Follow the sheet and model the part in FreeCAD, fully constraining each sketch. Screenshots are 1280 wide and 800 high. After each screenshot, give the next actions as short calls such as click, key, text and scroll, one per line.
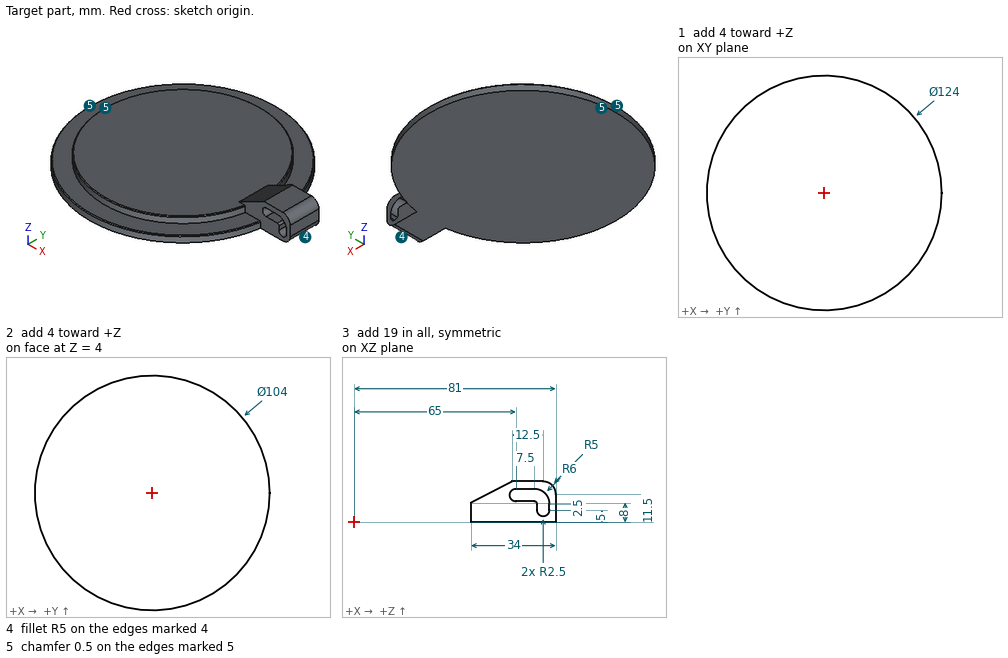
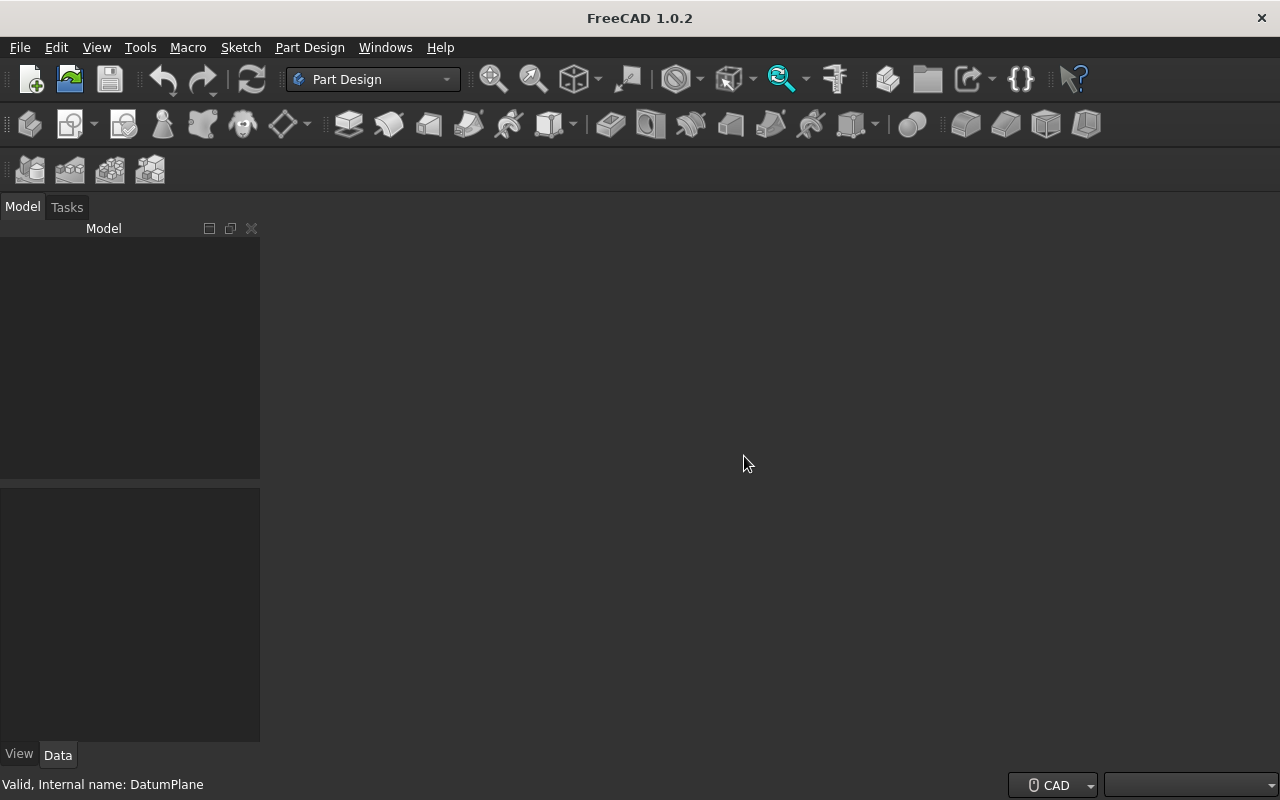
click(30, 80)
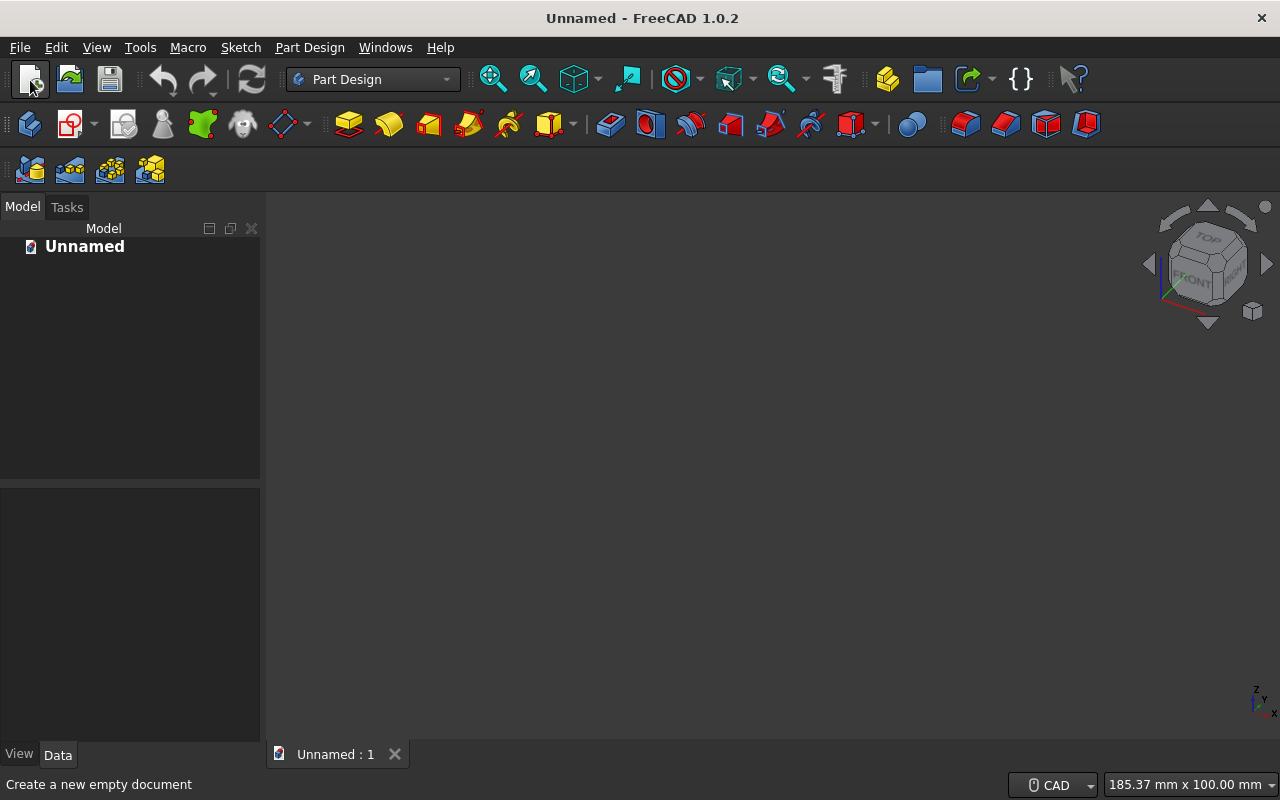
click(70, 124)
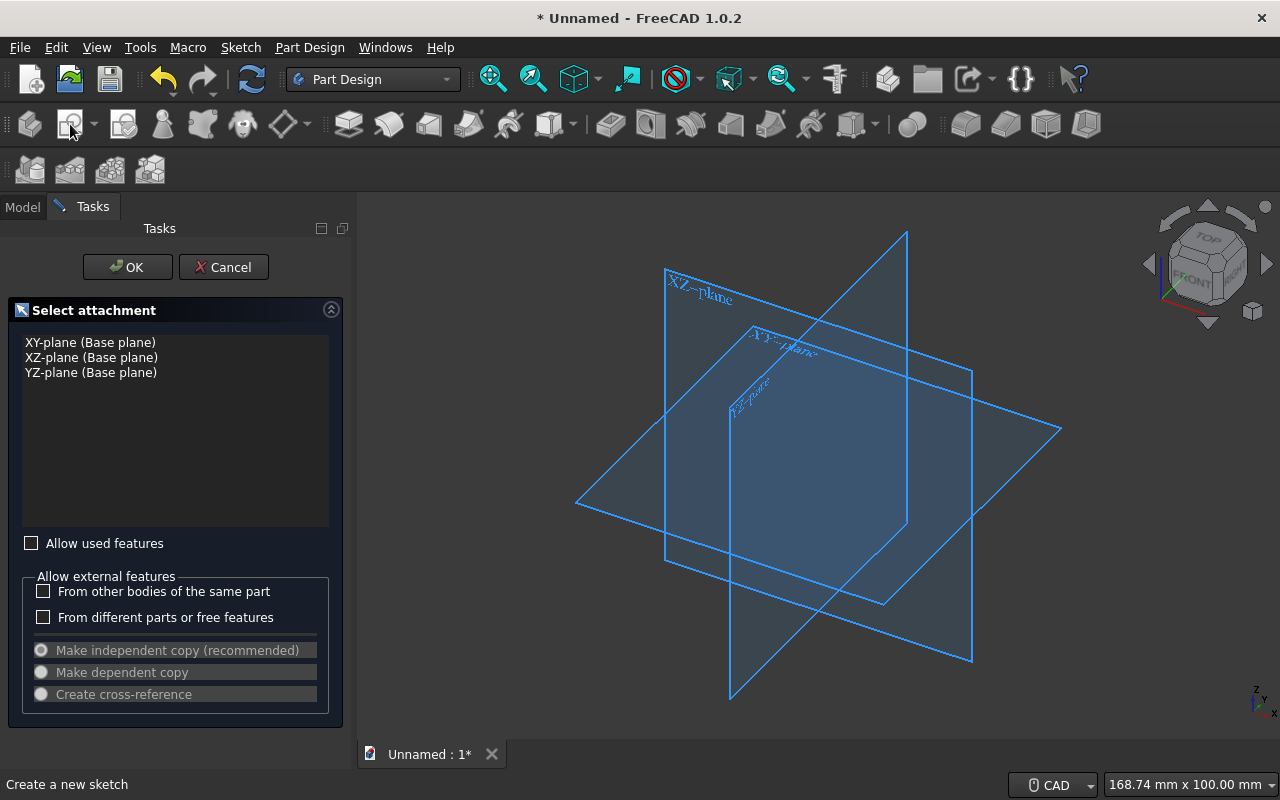
click(82, 342)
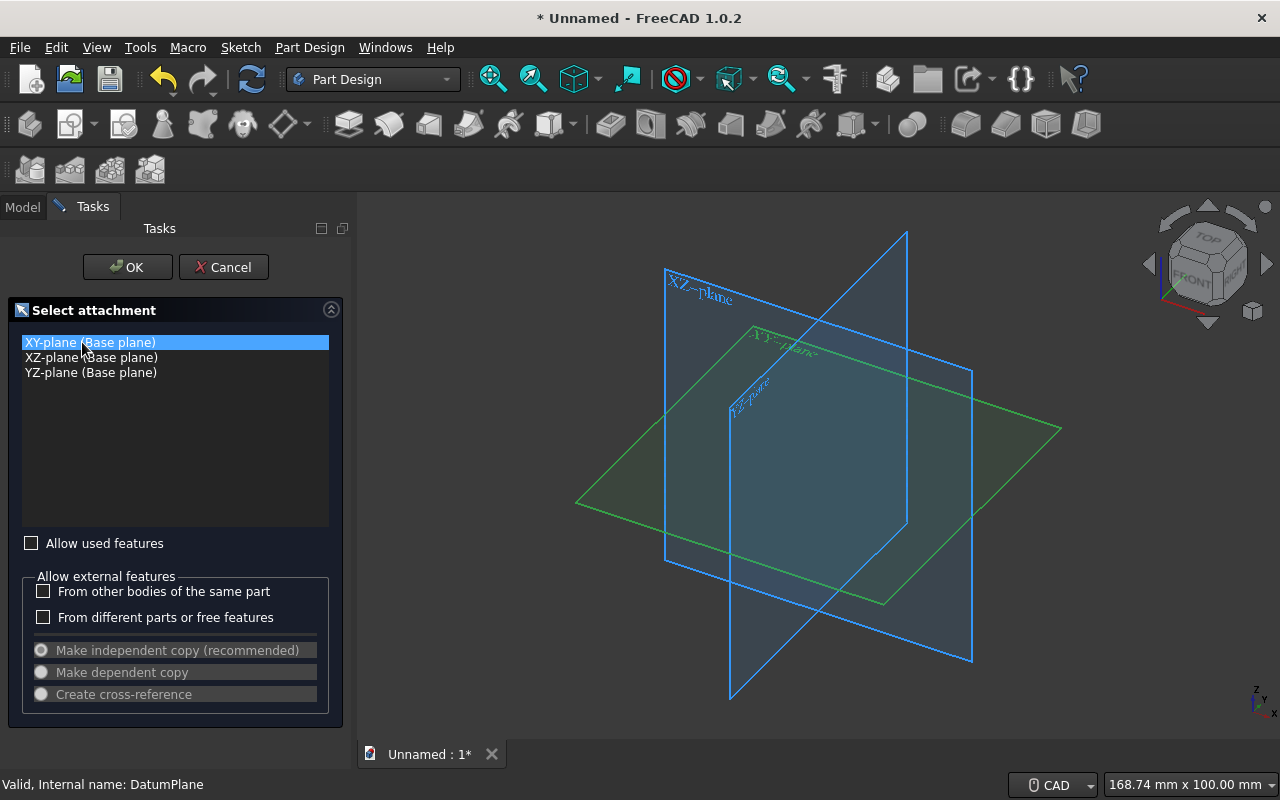
click(128, 267)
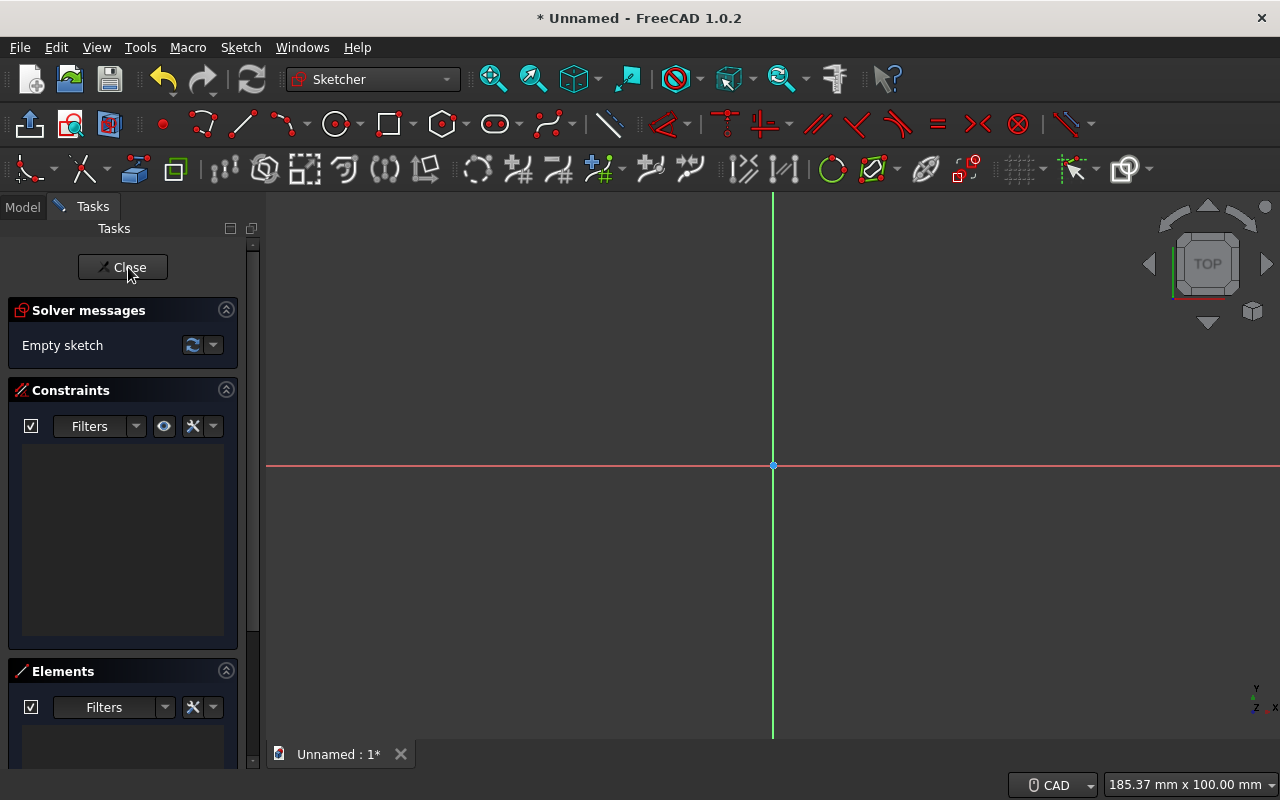
scroll(621, 466, down, 3)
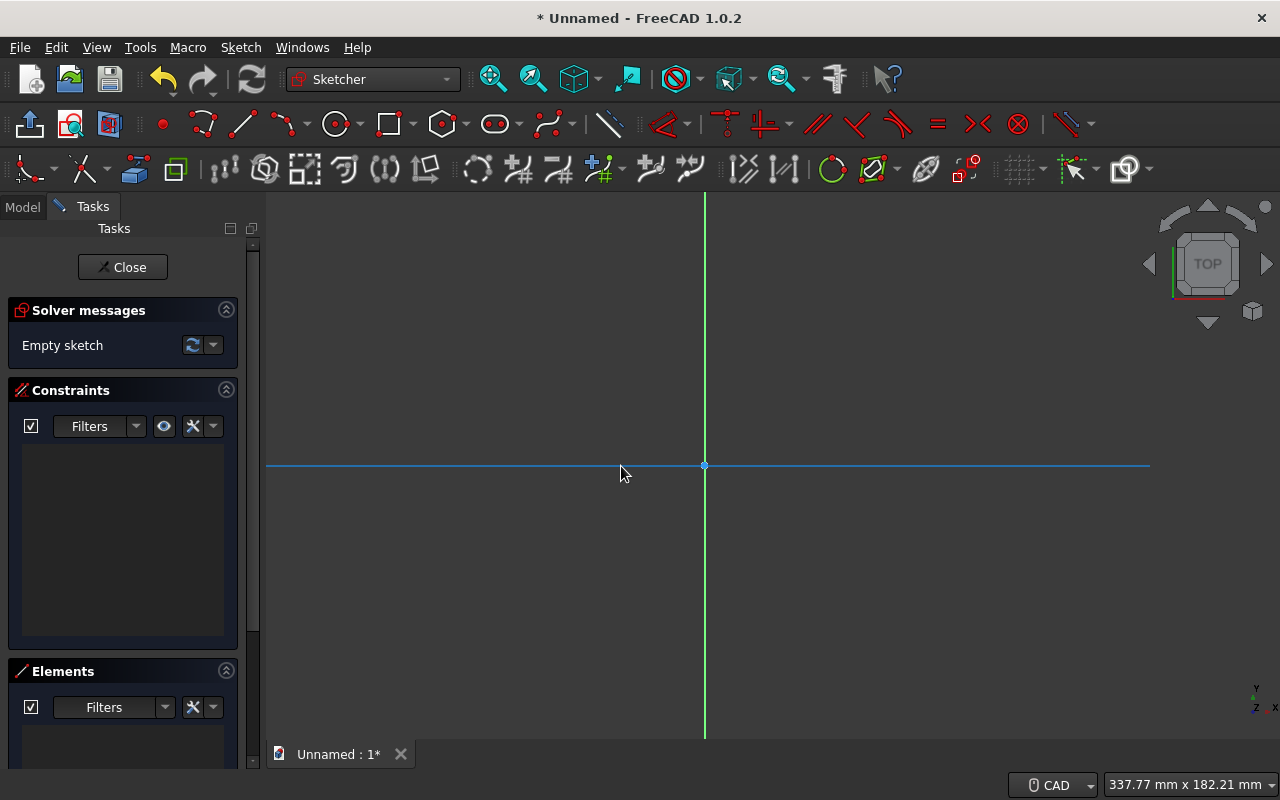
click(336, 124)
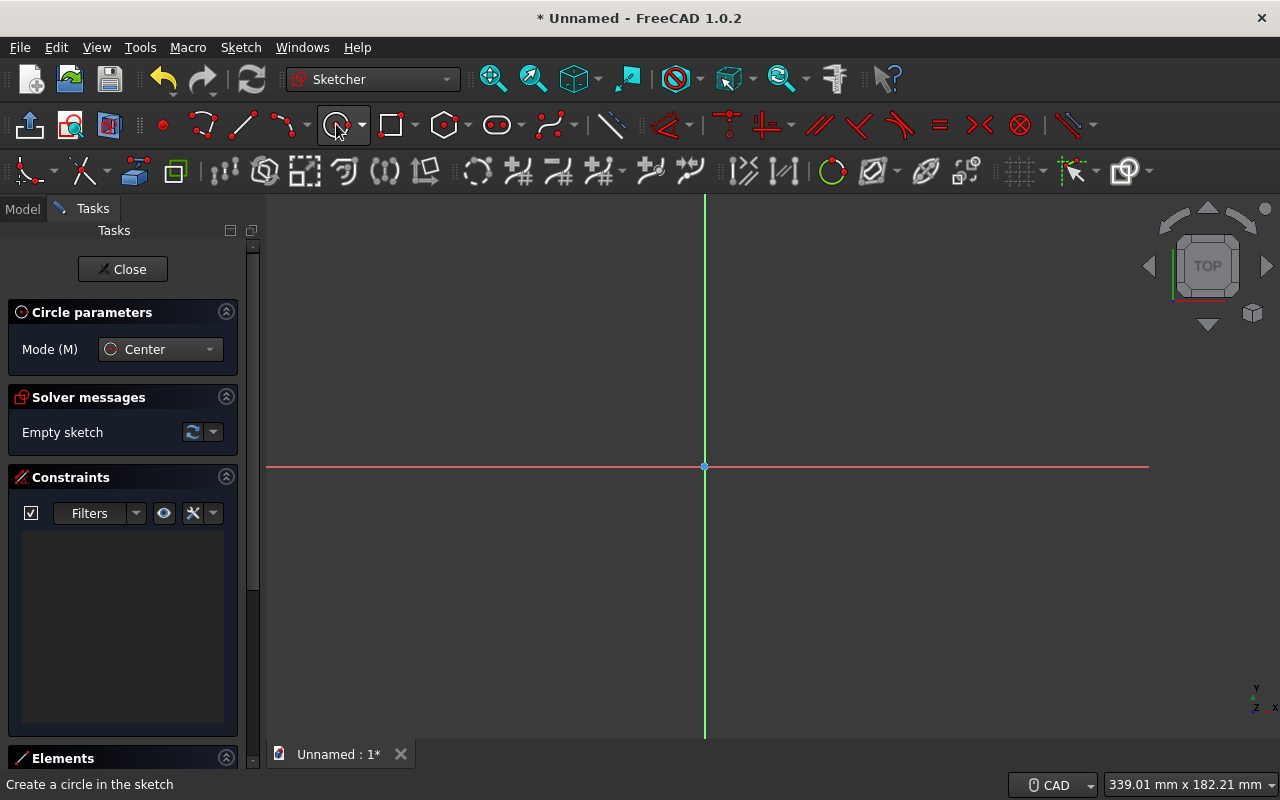
click(705, 467)
click(836, 336)
key(Escape)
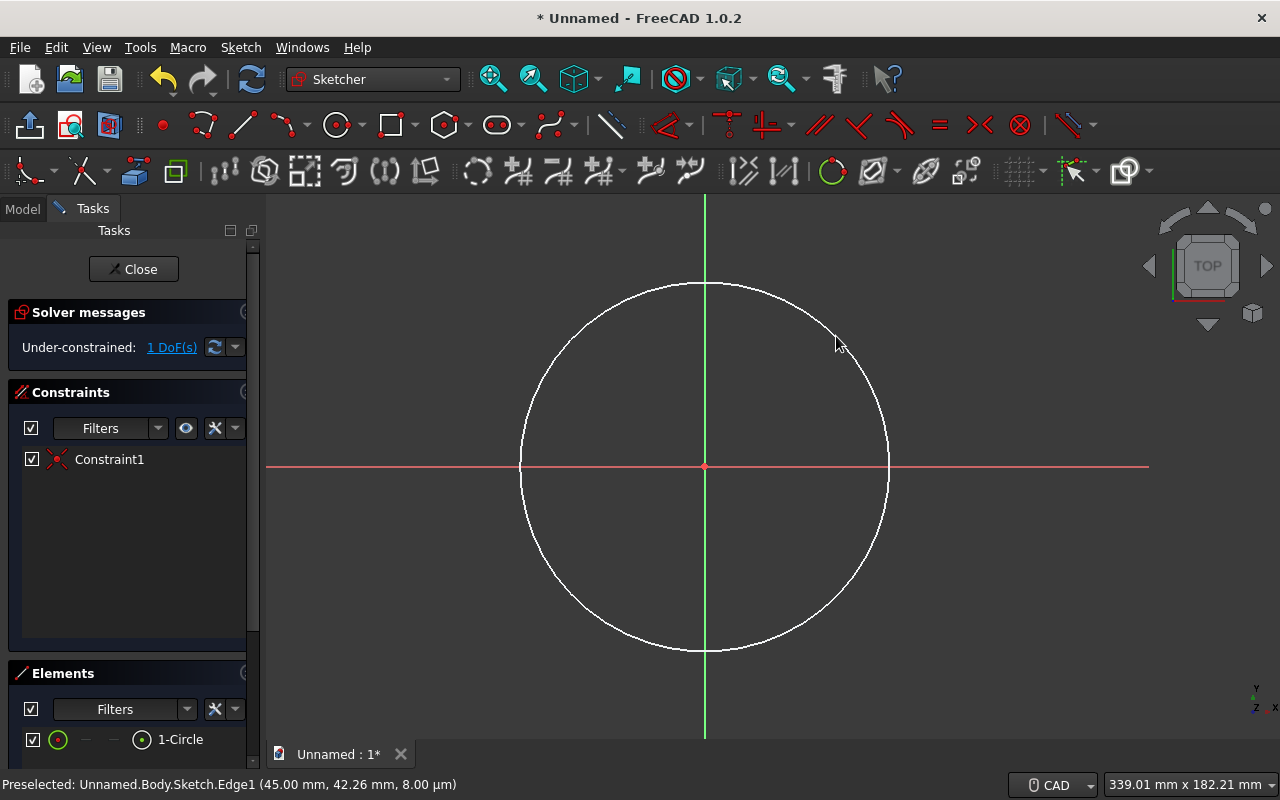
click(835, 336)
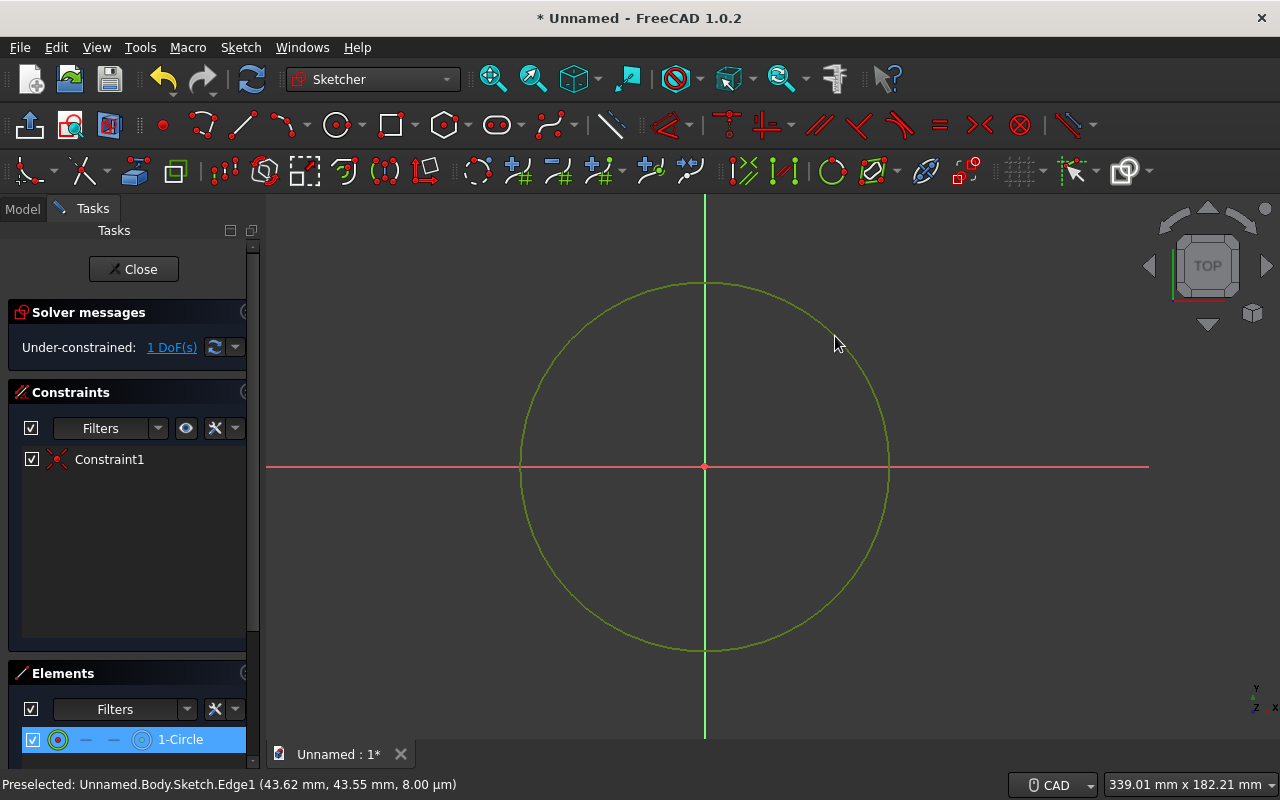
key(k)
key(o)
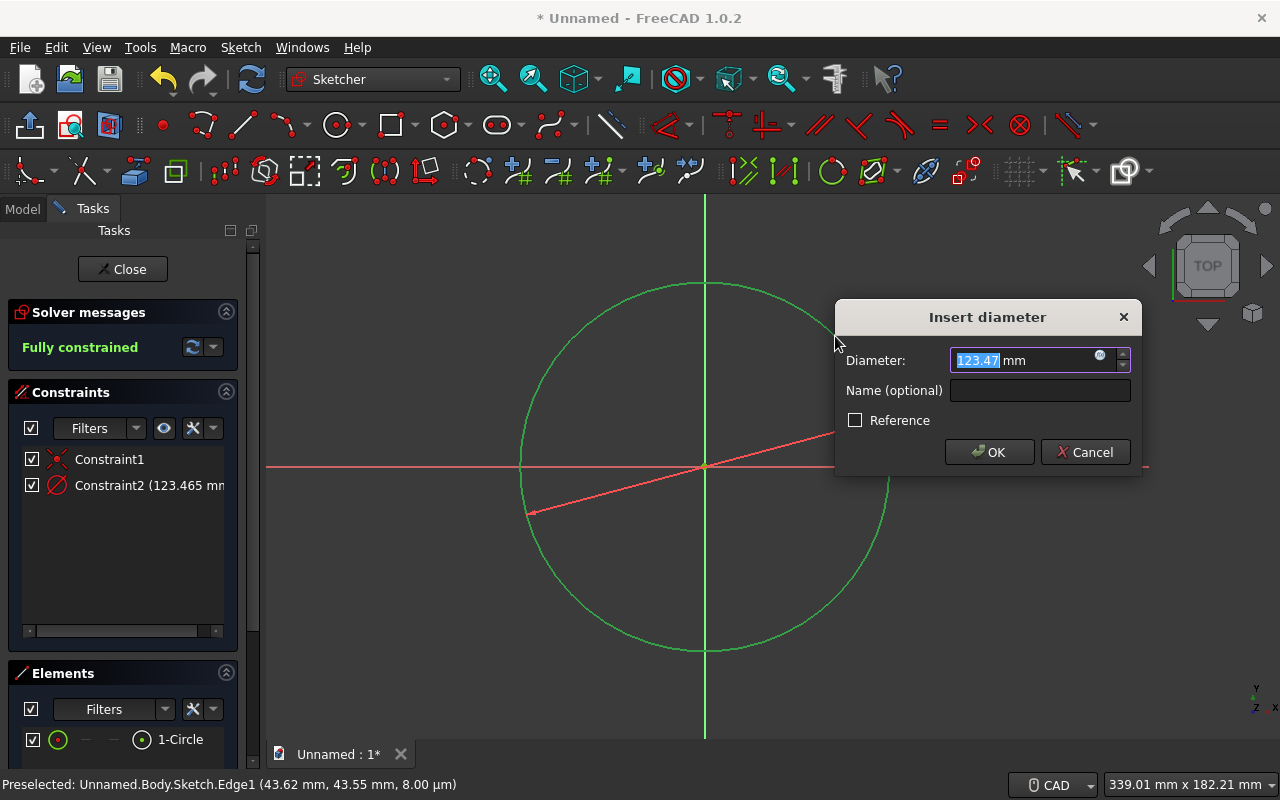
text(124)
key(Return)